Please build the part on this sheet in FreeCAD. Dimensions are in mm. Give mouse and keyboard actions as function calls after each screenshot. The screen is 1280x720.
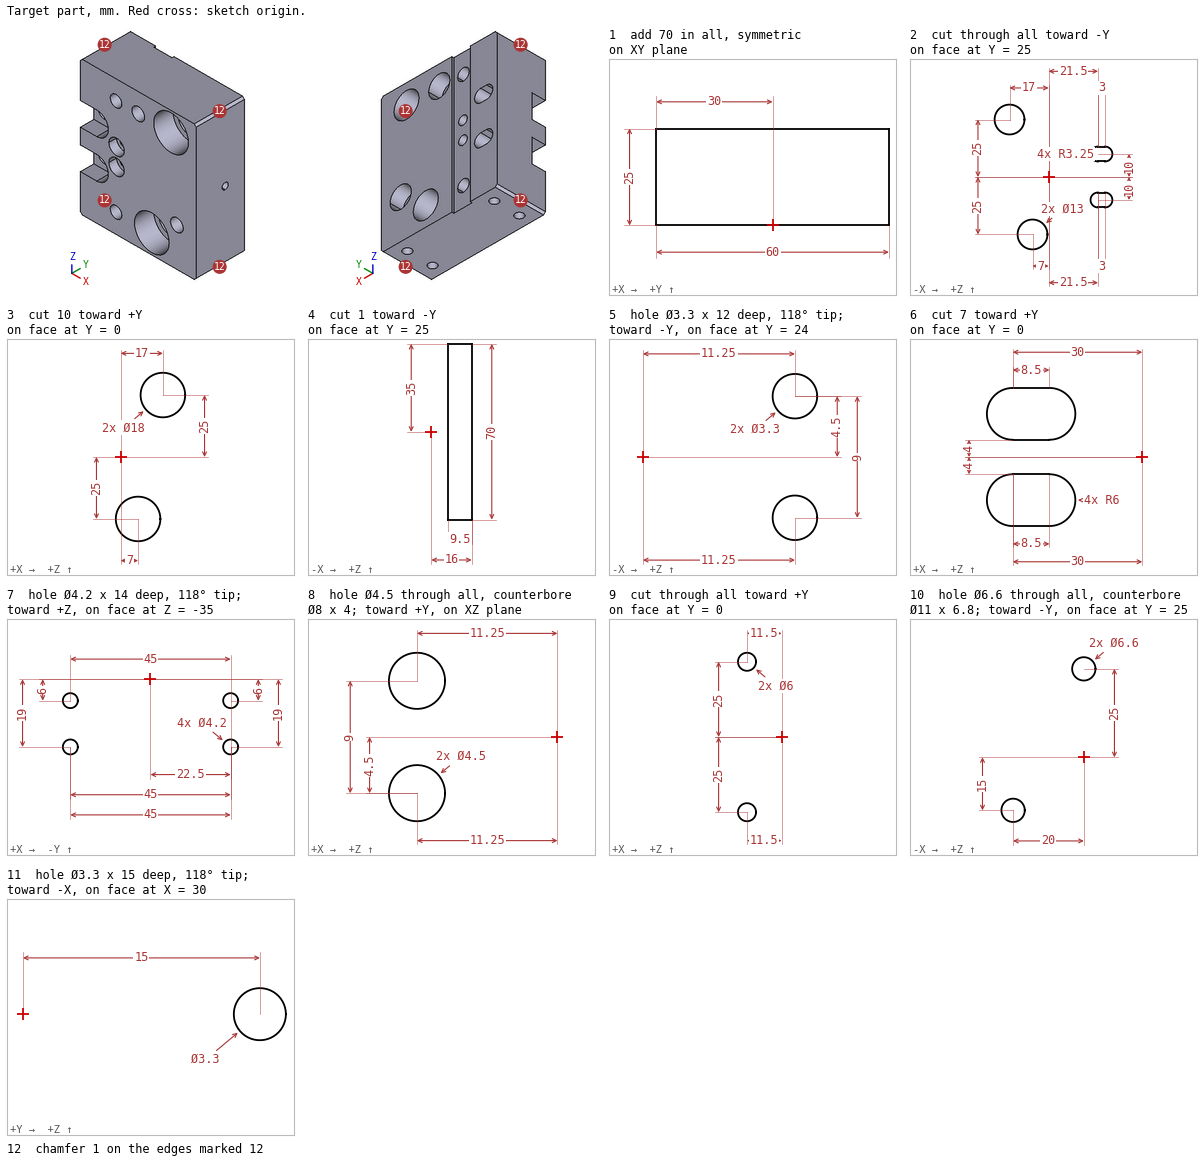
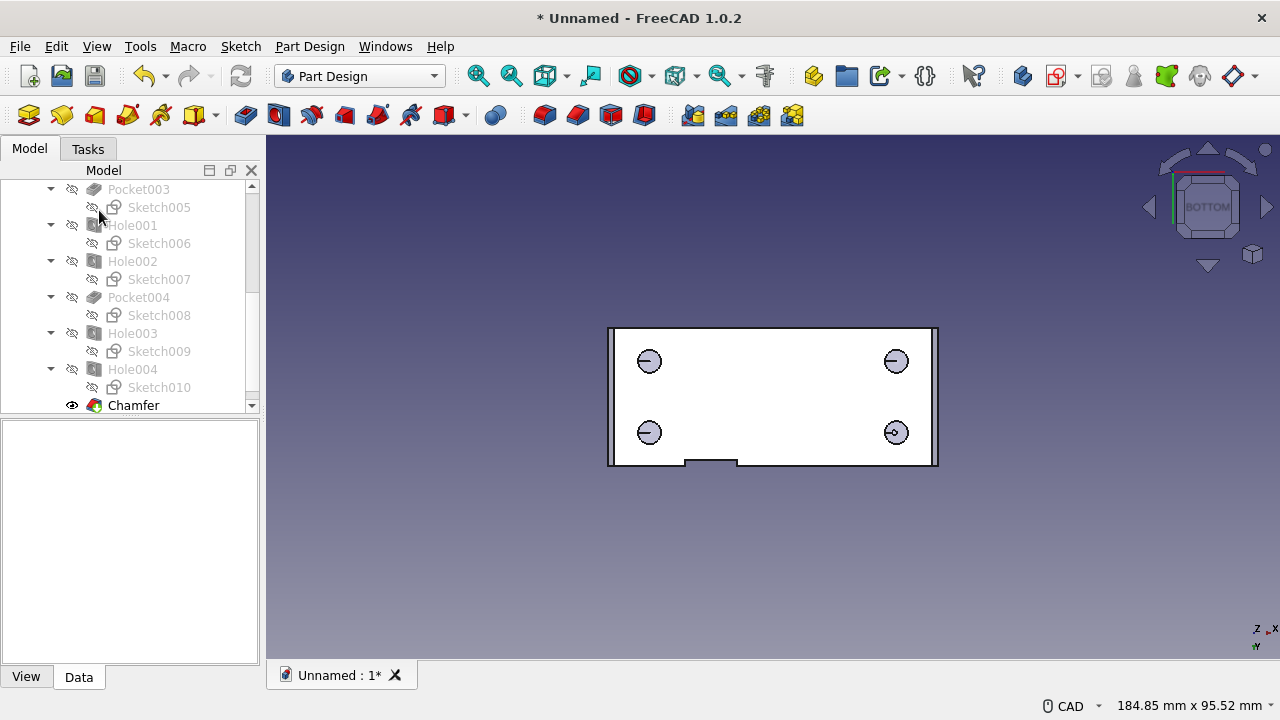
key(0)